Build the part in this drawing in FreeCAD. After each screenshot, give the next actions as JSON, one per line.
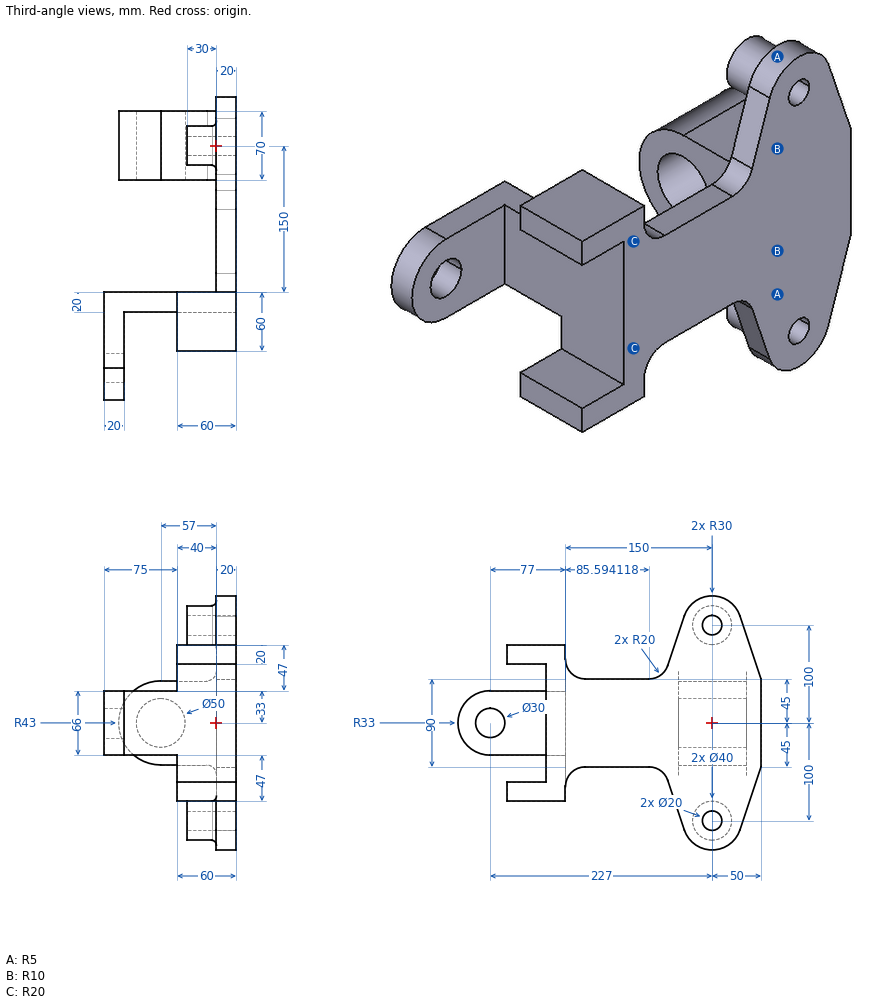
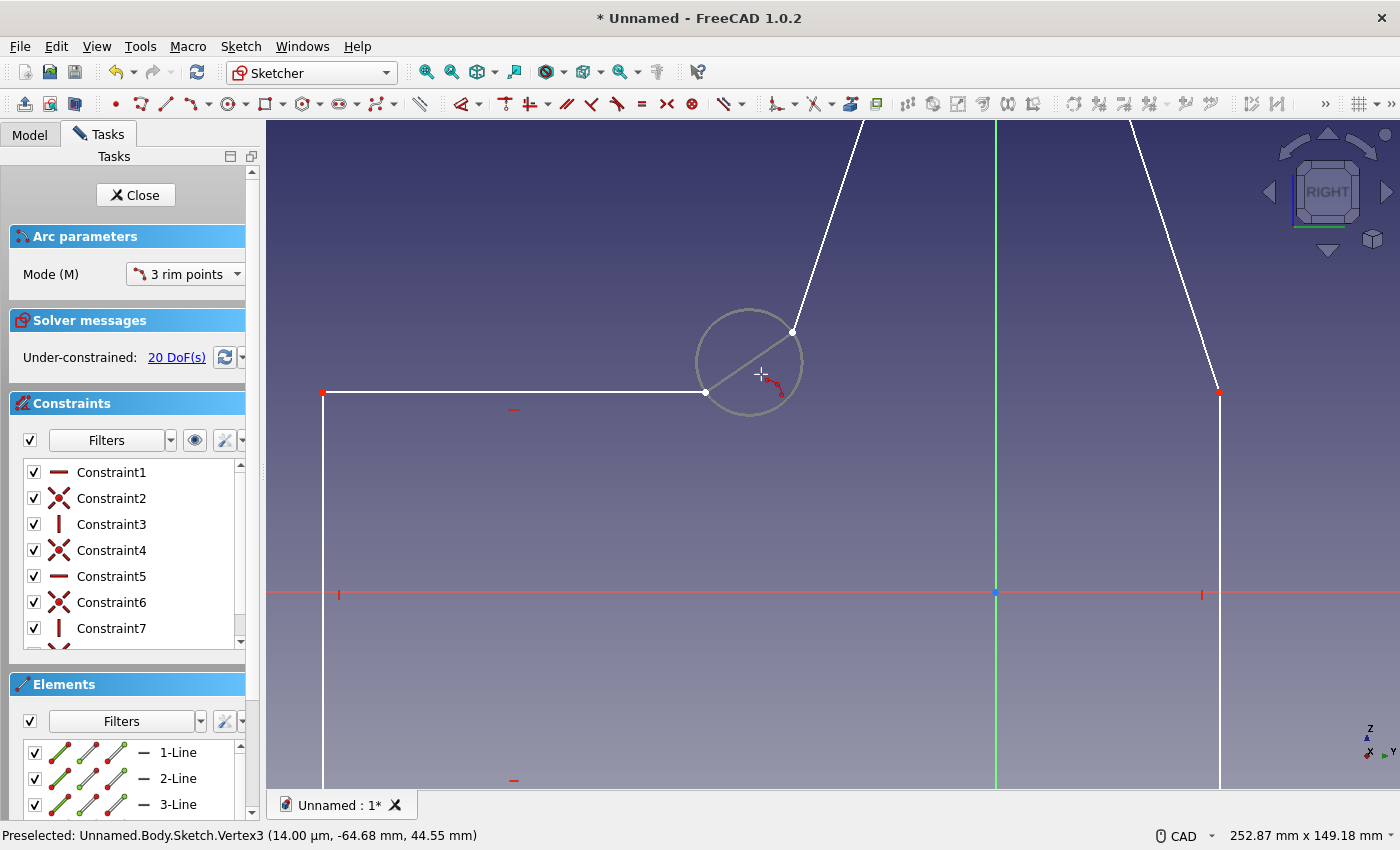
{"action": "left_click", "coordinate": [760, 373]}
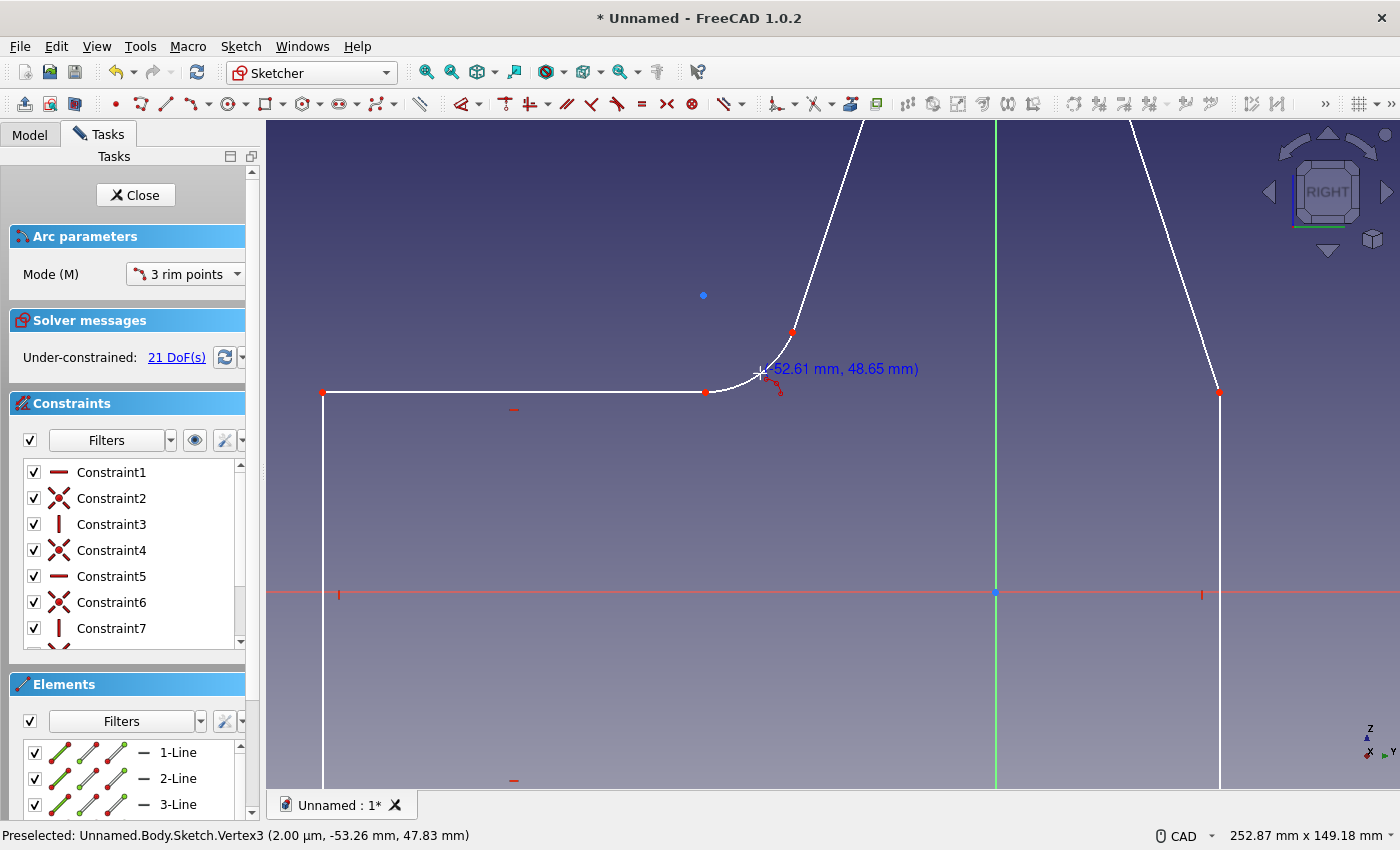
{"action": "scroll", "coordinate": [760, 374], "scroll_direction": "down", "scroll_amount": 5}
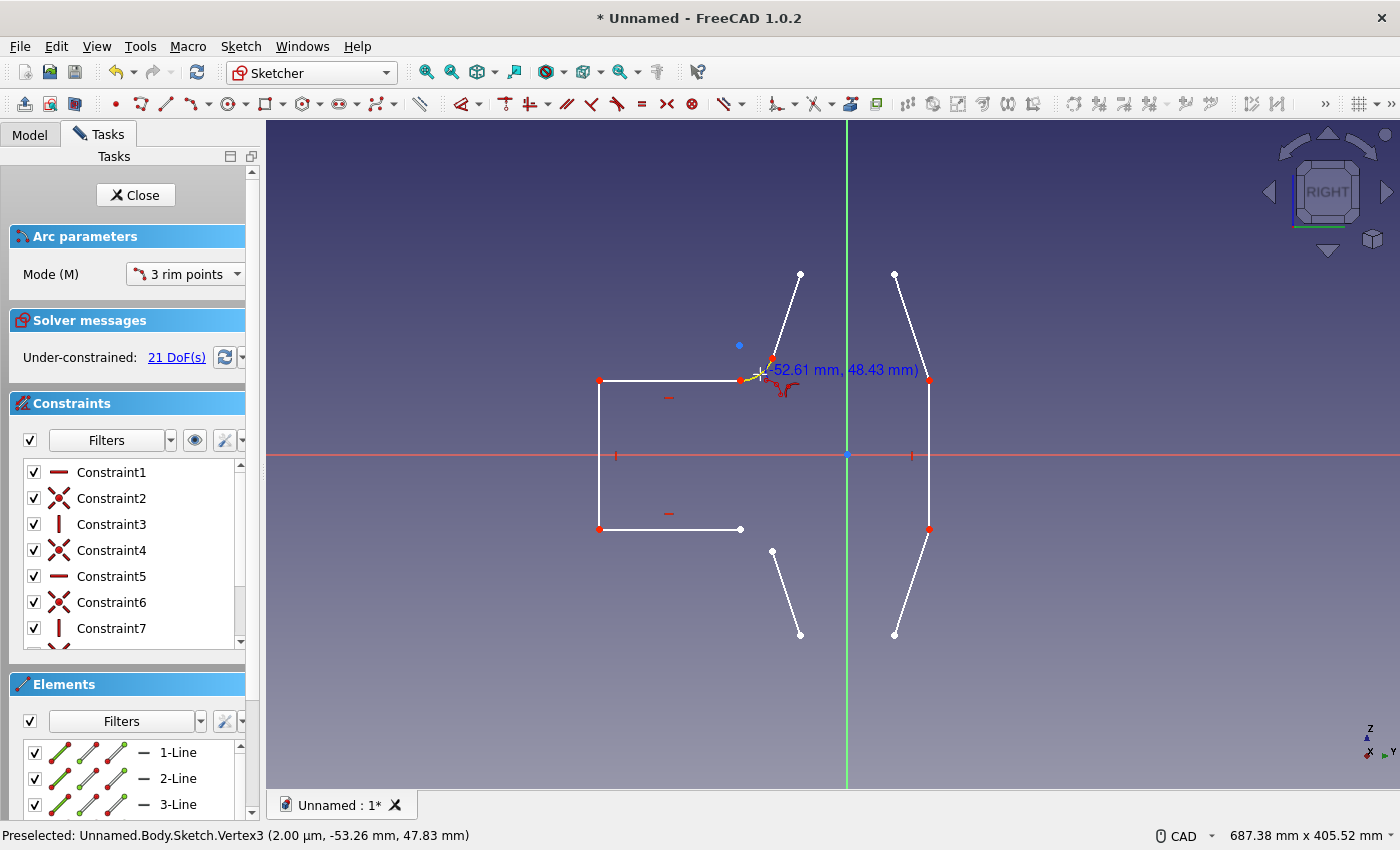
{"action": "left_click", "coordinate": [740, 530]}
{"action": "left_click", "coordinate": [772, 552]}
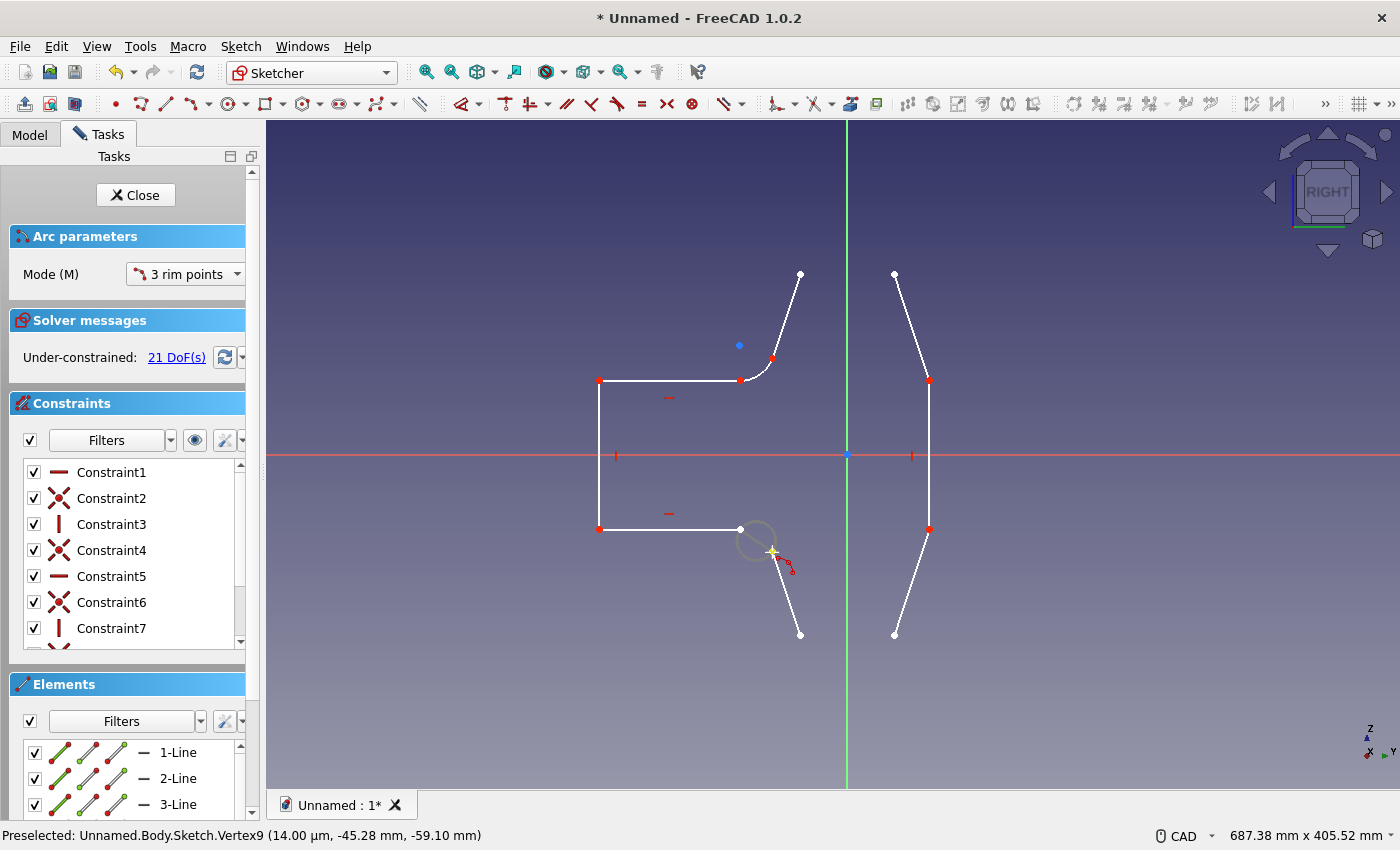
{"action": "scroll", "coordinate": [760, 535], "scroll_direction": "up", "scroll_amount": 5}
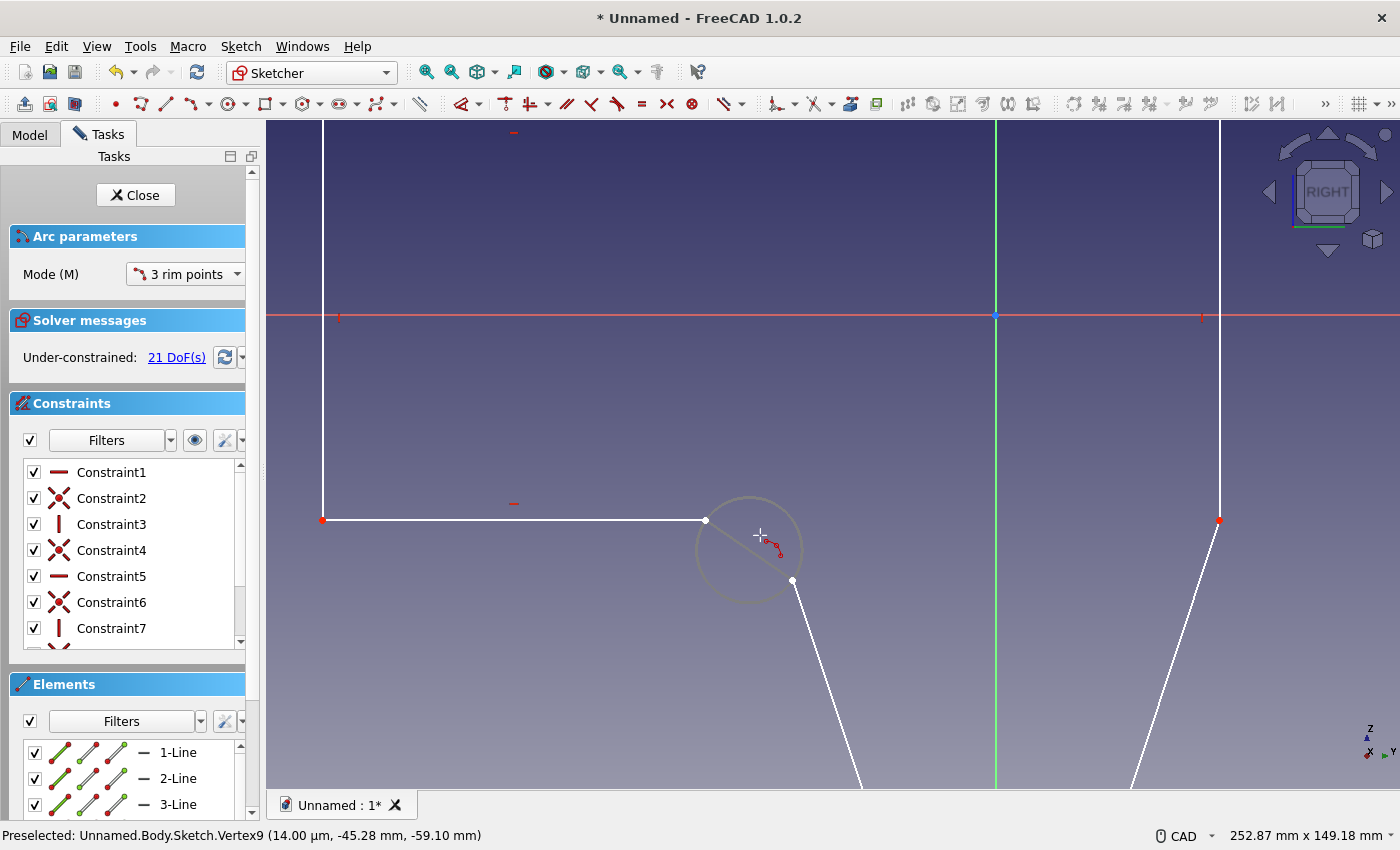
{"action": "left_click", "coordinate": [760, 534]}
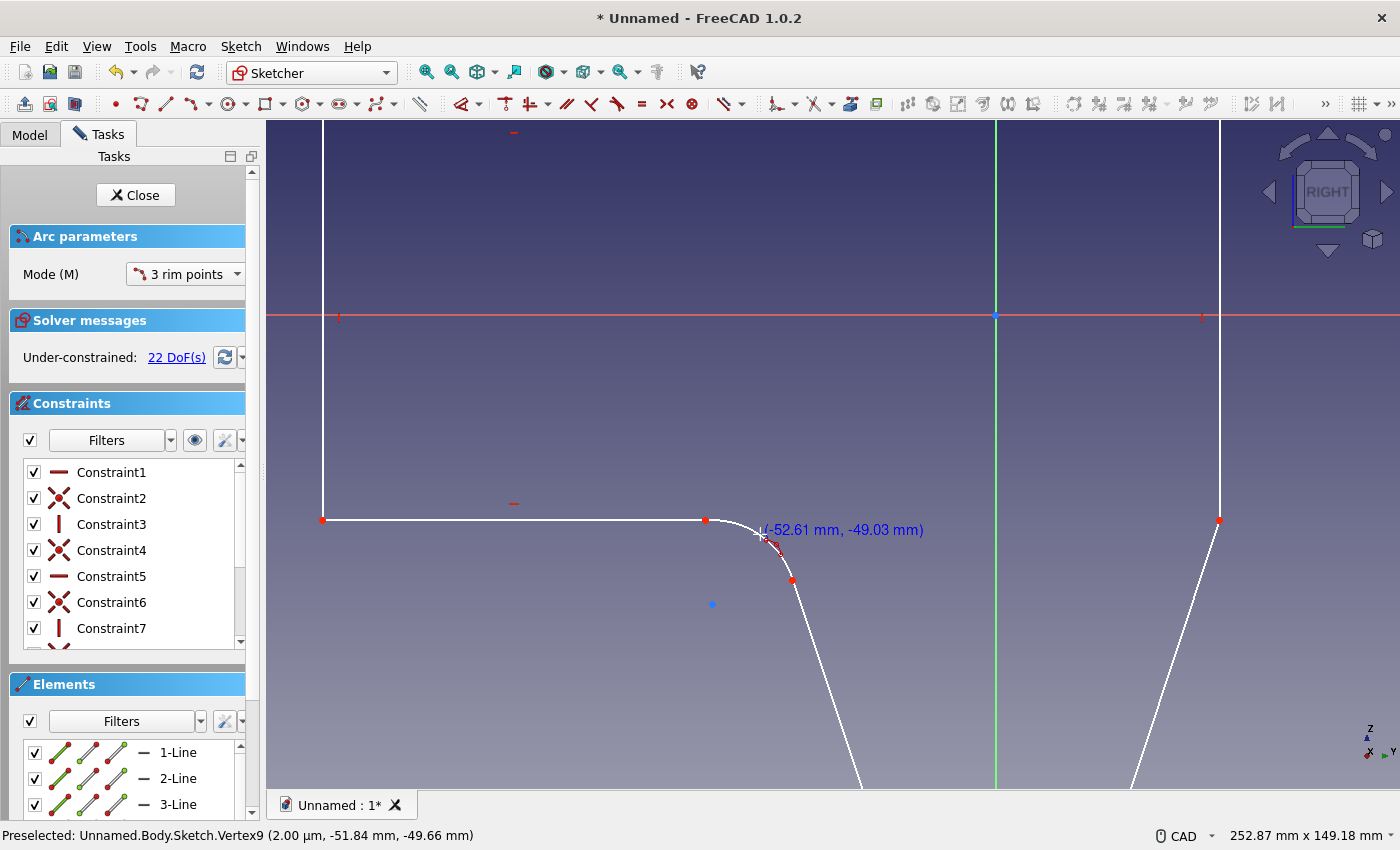
{"action": "scroll", "coordinate": [760, 536], "scroll_direction": "down", "scroll_amount": 5}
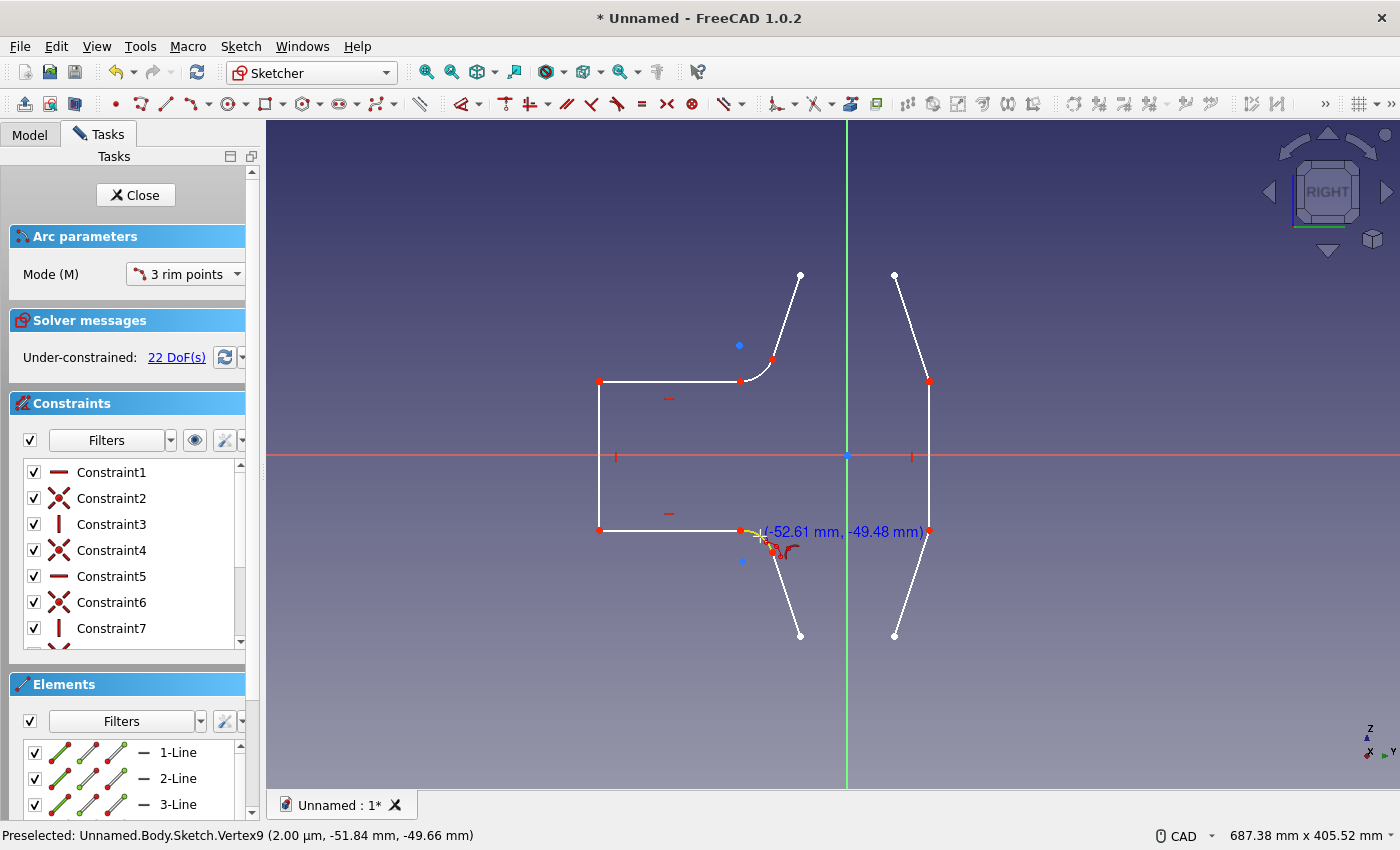
{"action": "left_click", "coordinate": [800, 637]}
{"action": "left_click", "coordinate": [894, 637]}
{"action": "left_click", "coordinate": [823, 664]}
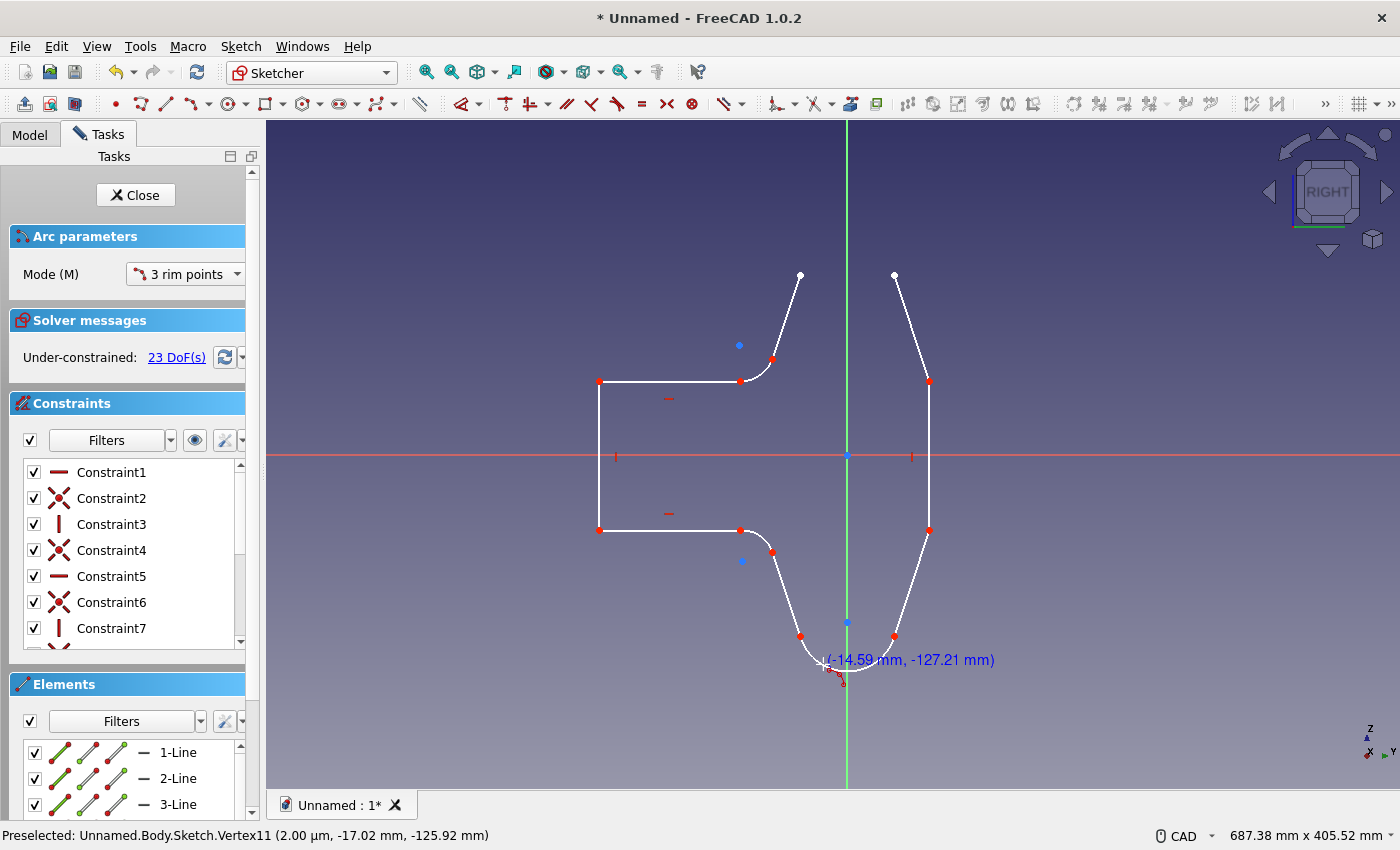
{"action": "left_click", "coordinate": [894, 276]}
{"action": "left_click", "coordinate": [800, 276]}
{"action": "left_click", "coordinate": [871, 247]}
{"action": "key", "text": "Escape"}